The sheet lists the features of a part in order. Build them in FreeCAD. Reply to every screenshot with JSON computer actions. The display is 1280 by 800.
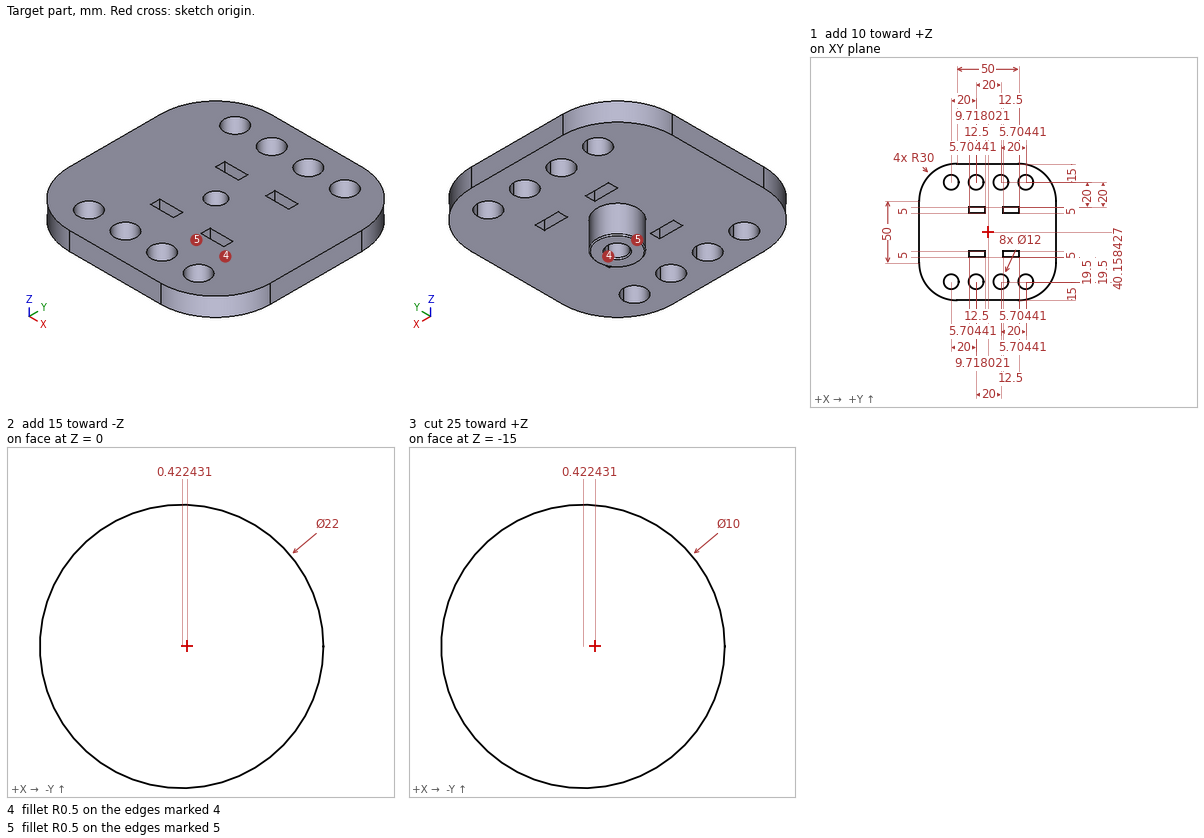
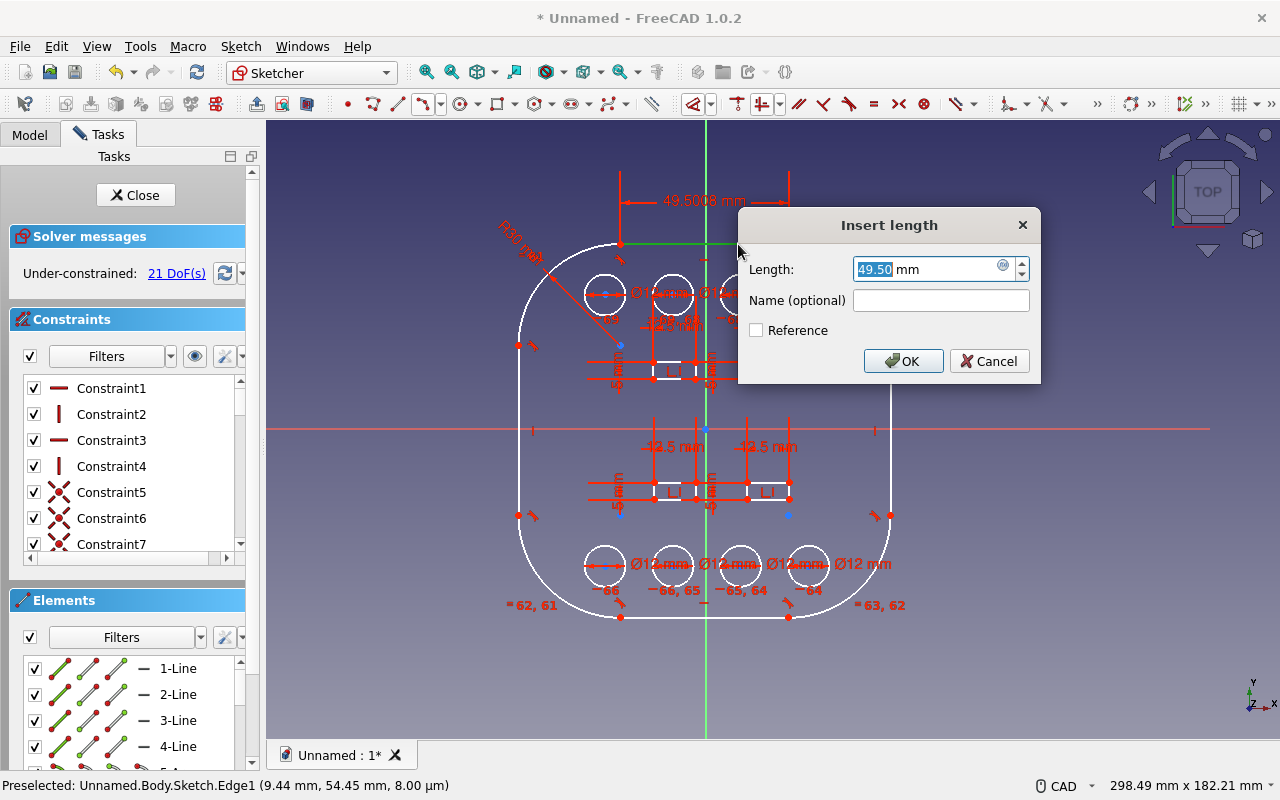
{"action": "type", "text": "50"}
{"action": "key", "text": "Return"}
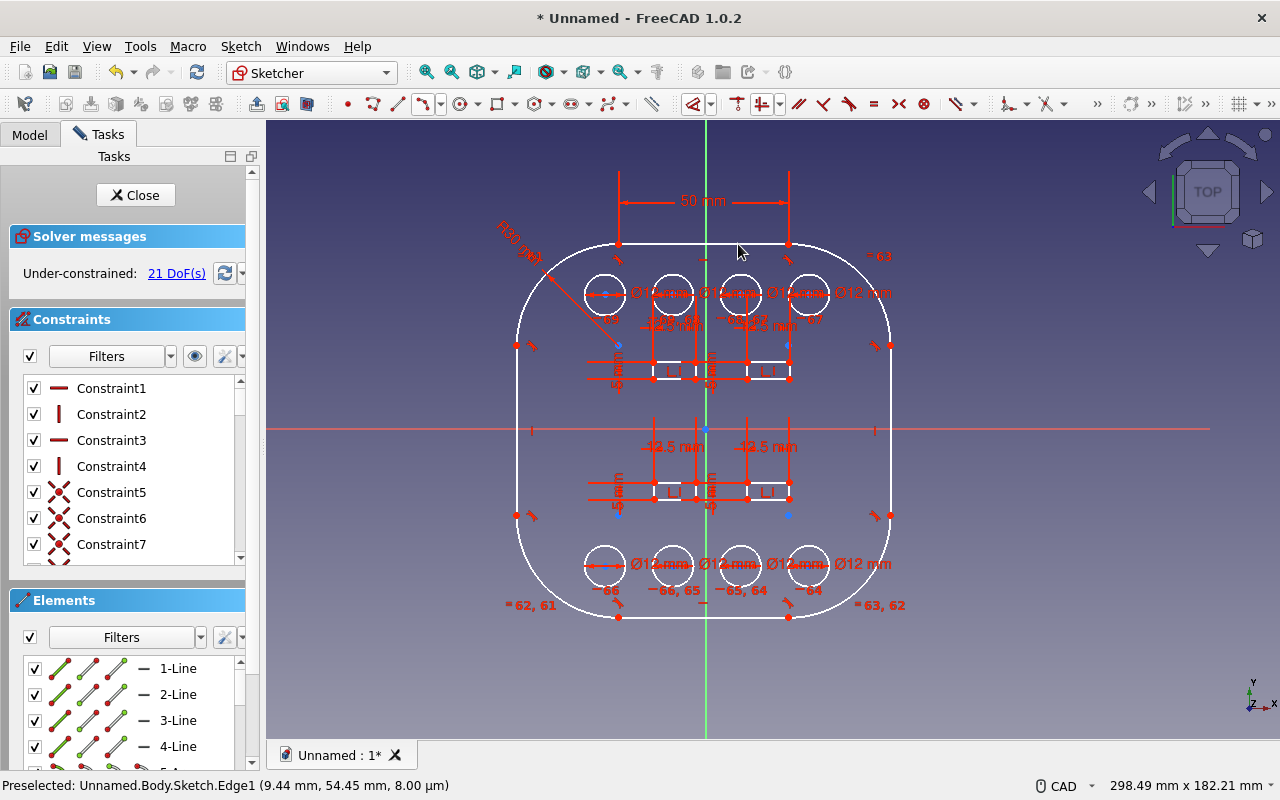
{"action": "left_click", "coordinate": [517, 397]}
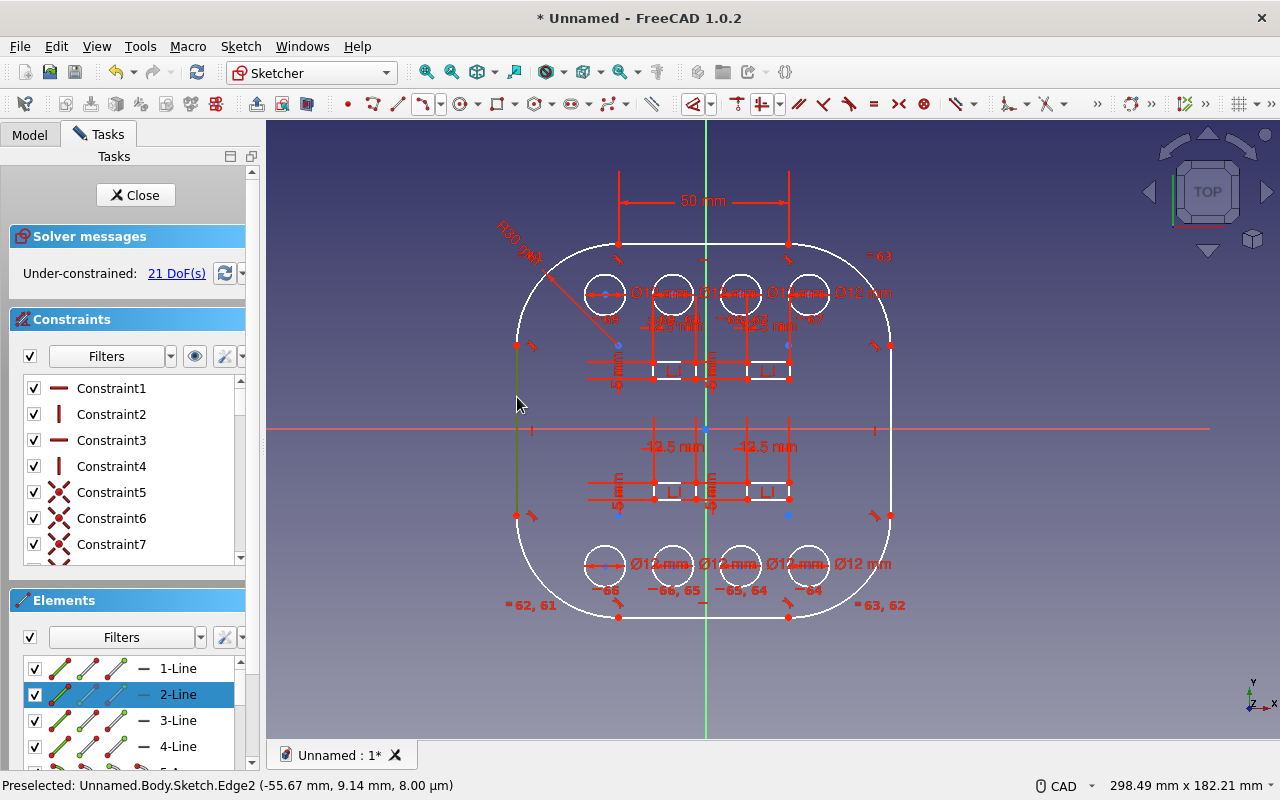
{"action": "key", "text": "i"}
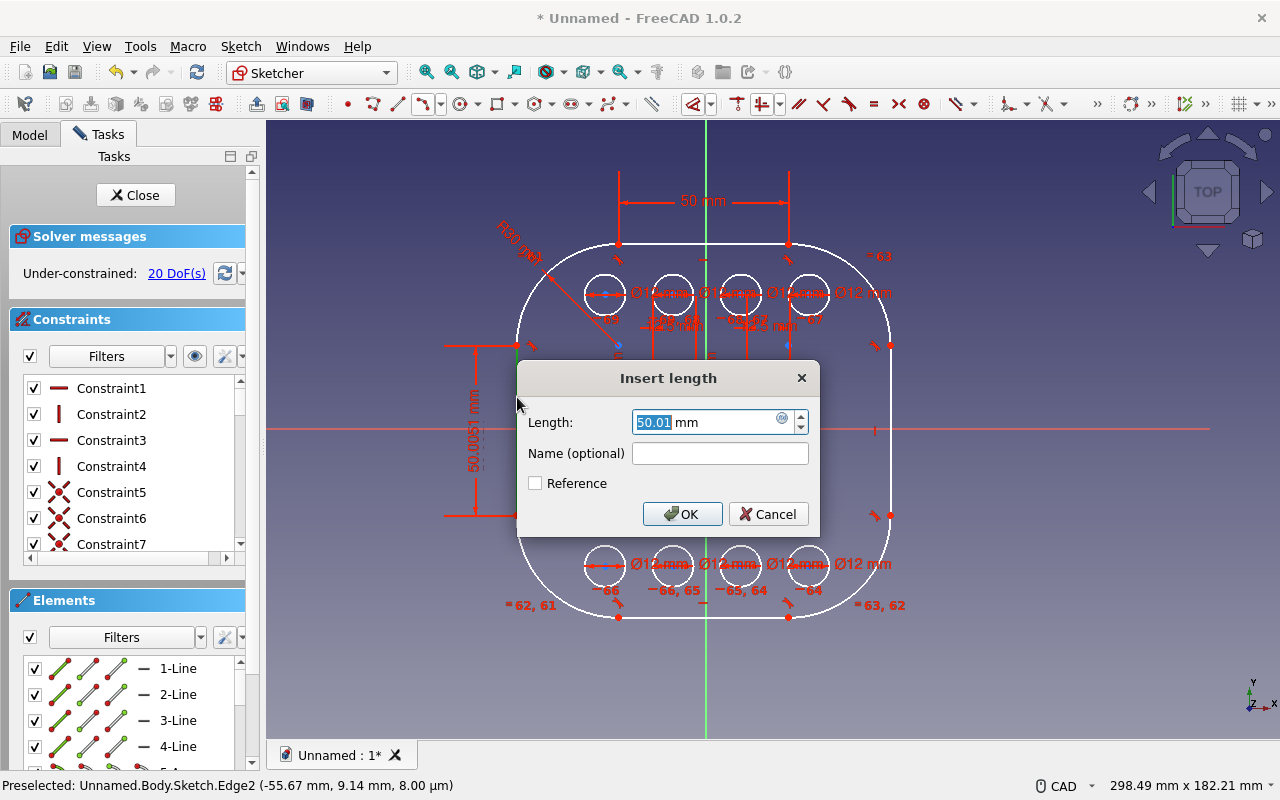
{"action": "type", "text": "50"}
{"action": "key", "text": "Return"}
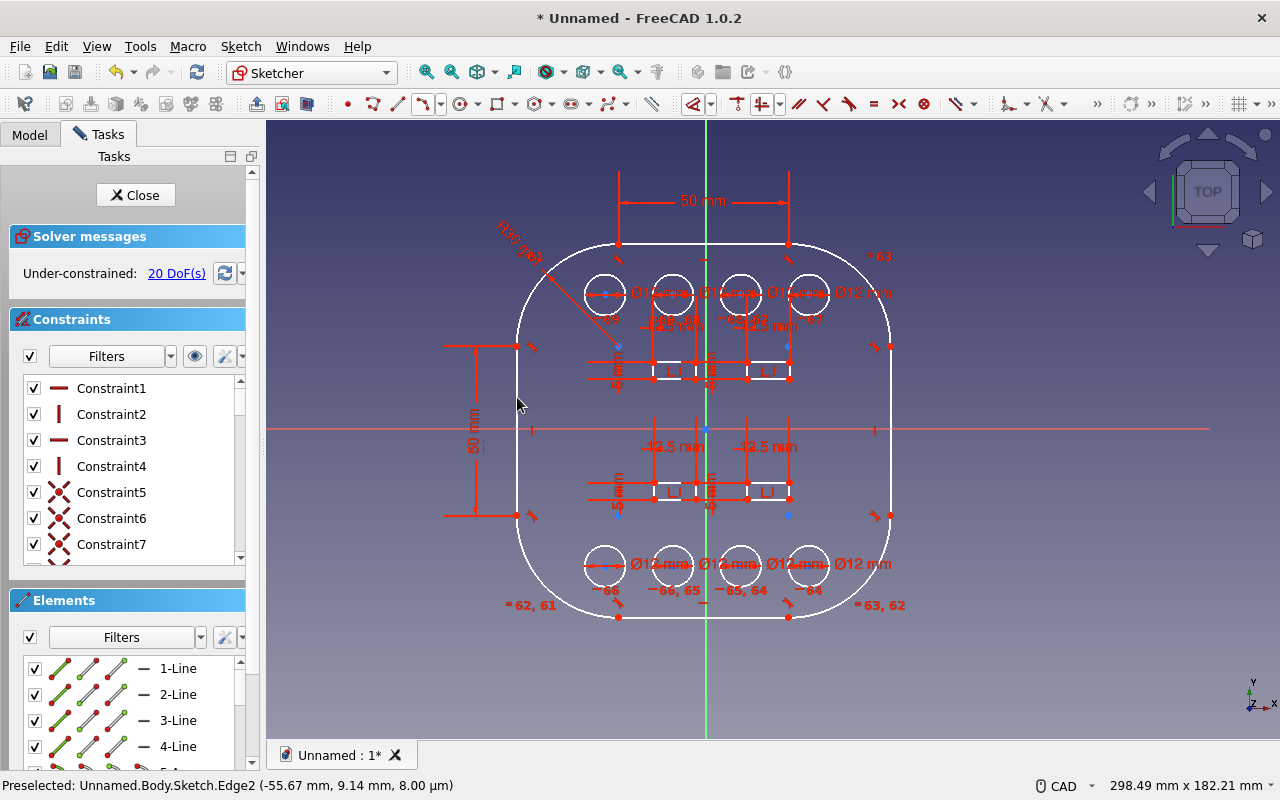
{"action": "left_click", "coordinate": [789, 618]}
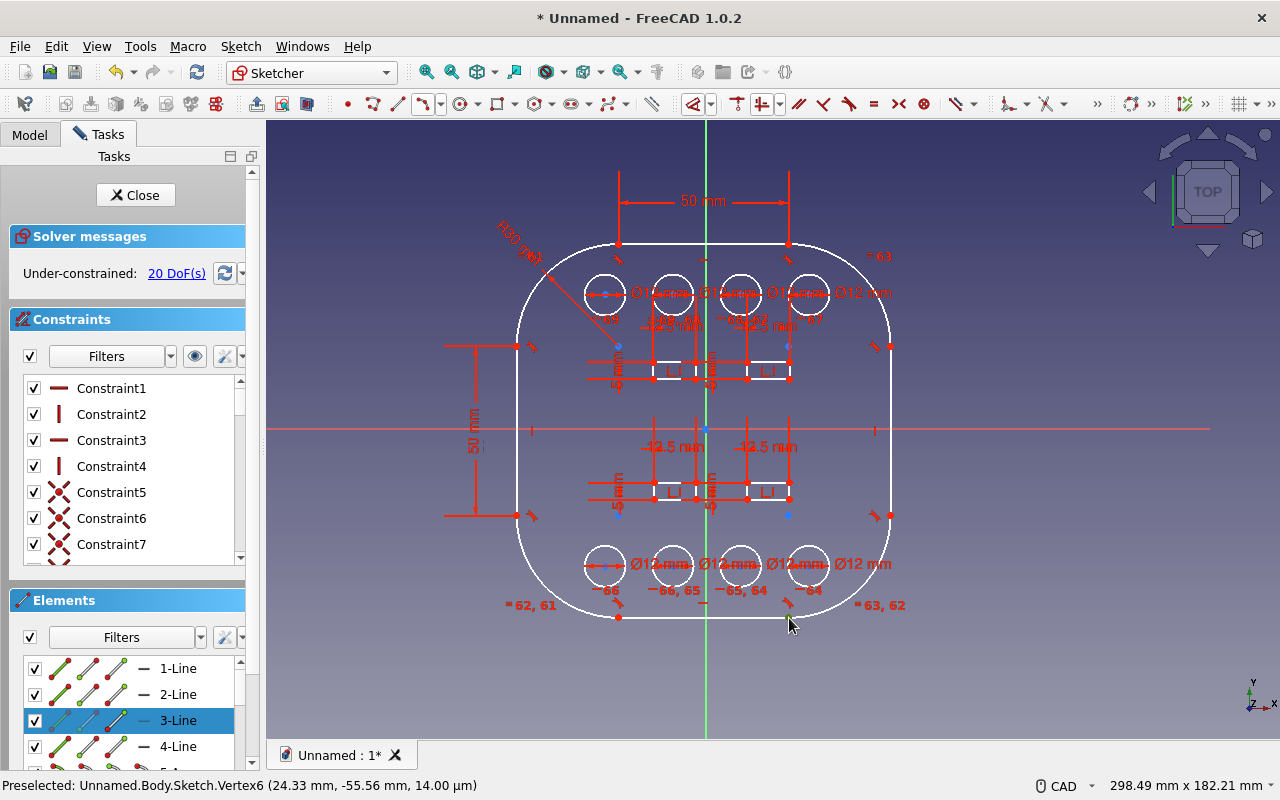
{"action": "left_click", "coordinate": [809, 566]}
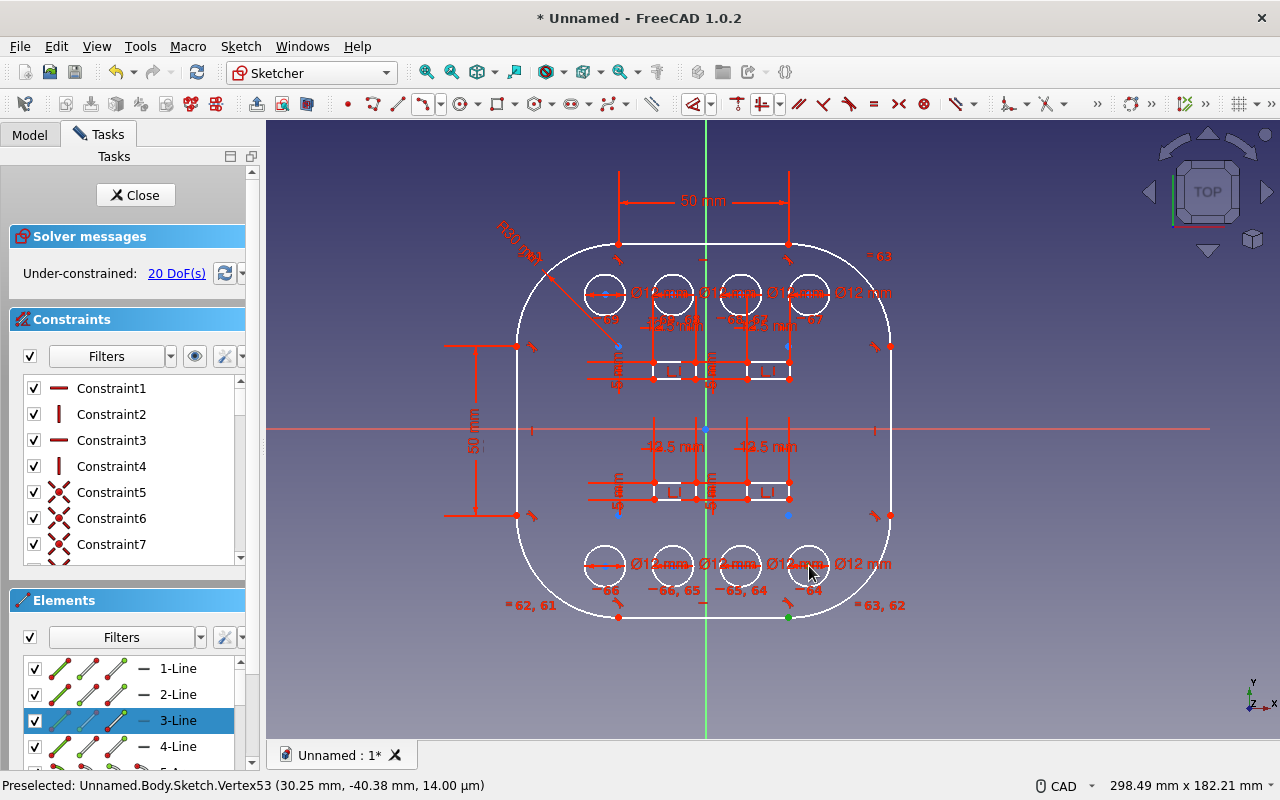
{"action": "key", "text": "i"}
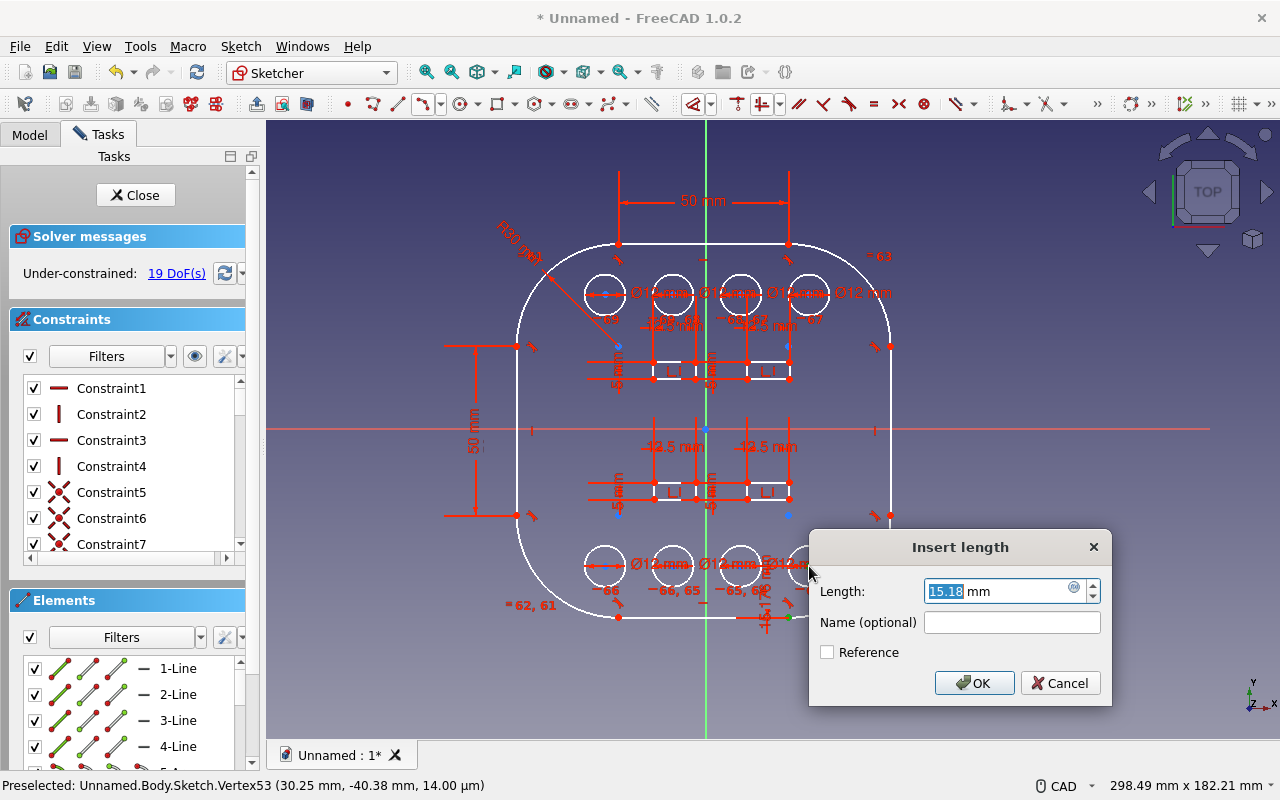
{"action": "type", "text": "15"}
{"action": "key", "text": "Return"}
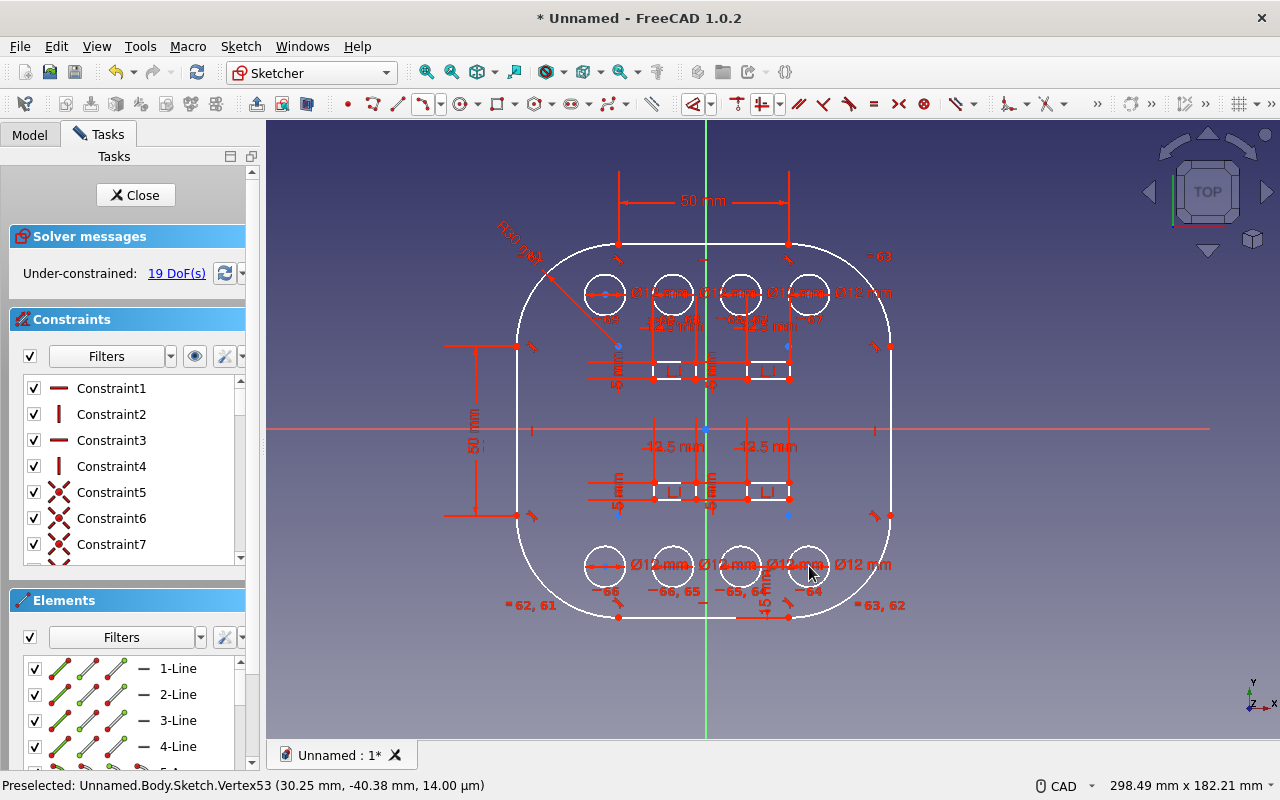
{"action": "left_click", "coordinate": [809, 567]}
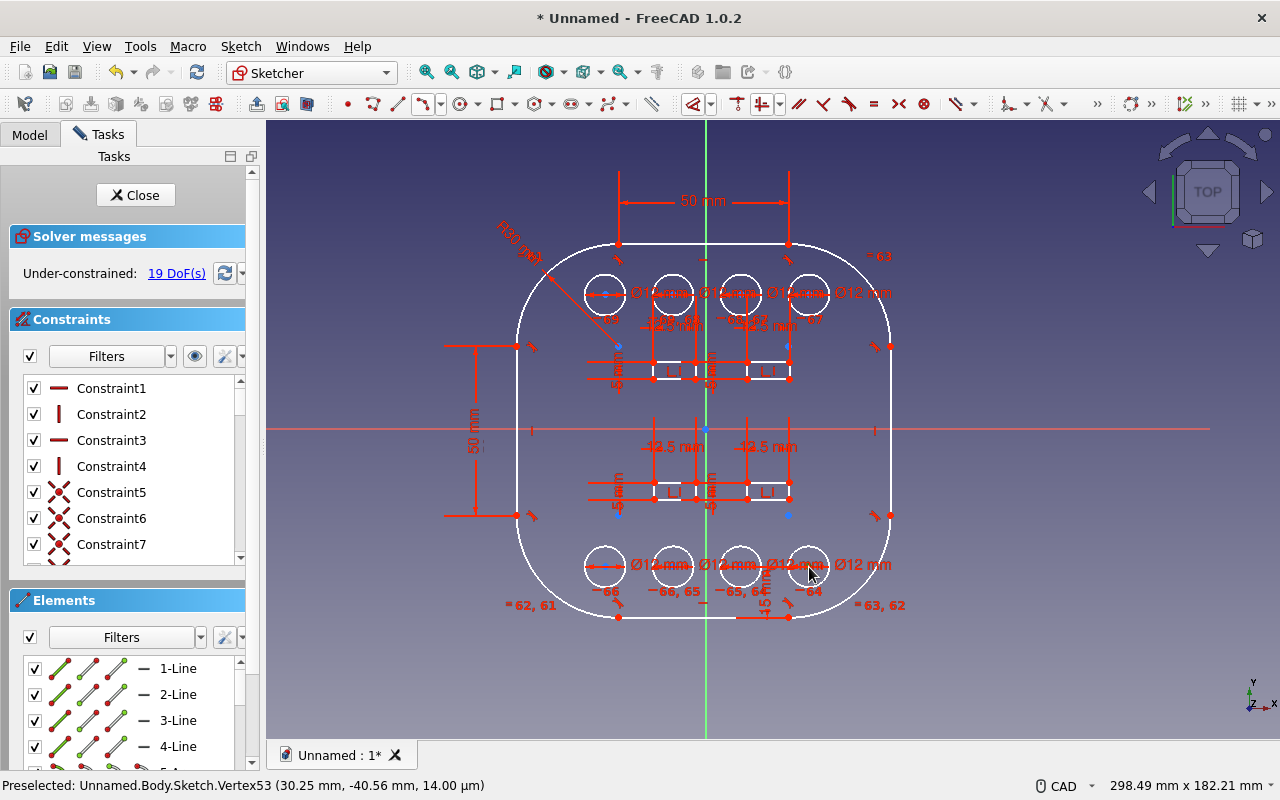
{"action": "left_click", "coordinate": [741, 567]}